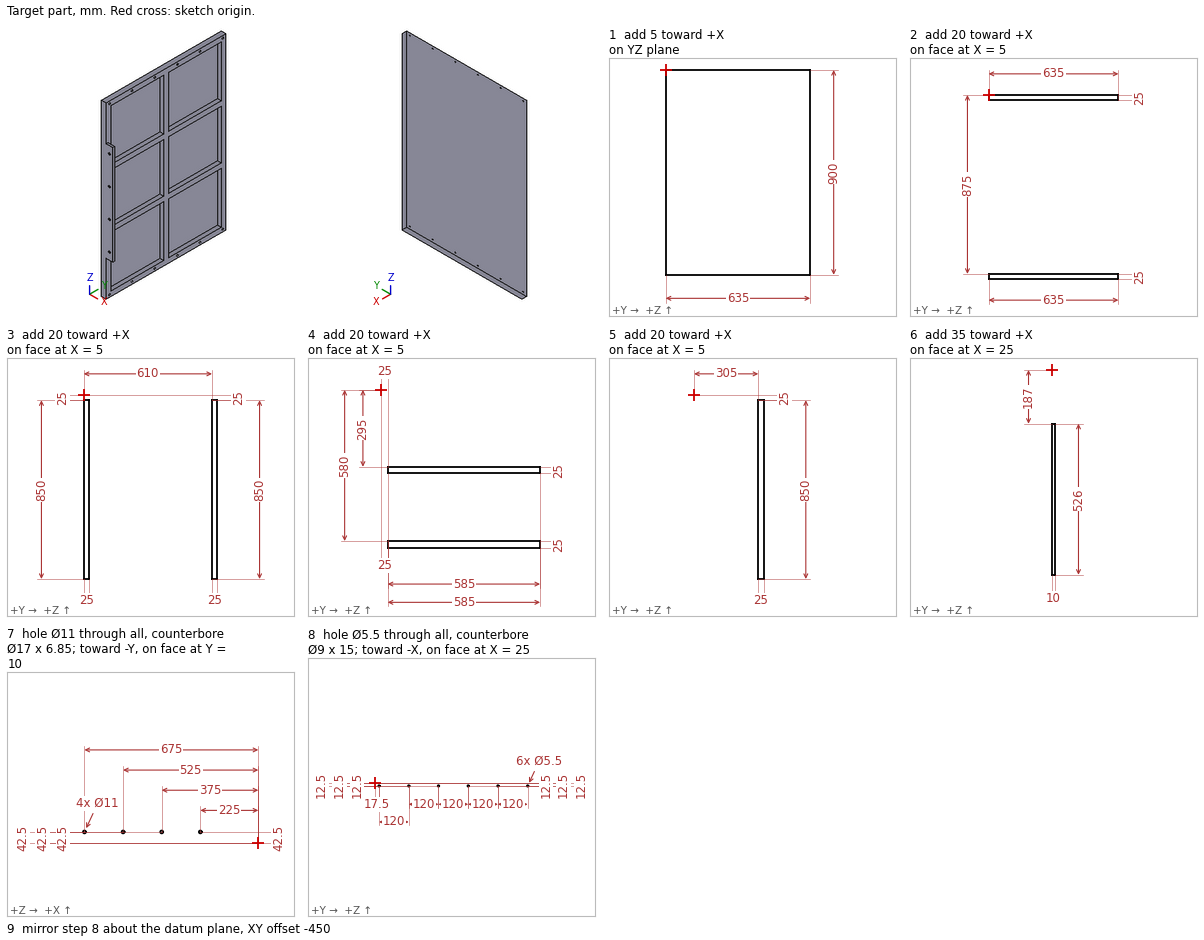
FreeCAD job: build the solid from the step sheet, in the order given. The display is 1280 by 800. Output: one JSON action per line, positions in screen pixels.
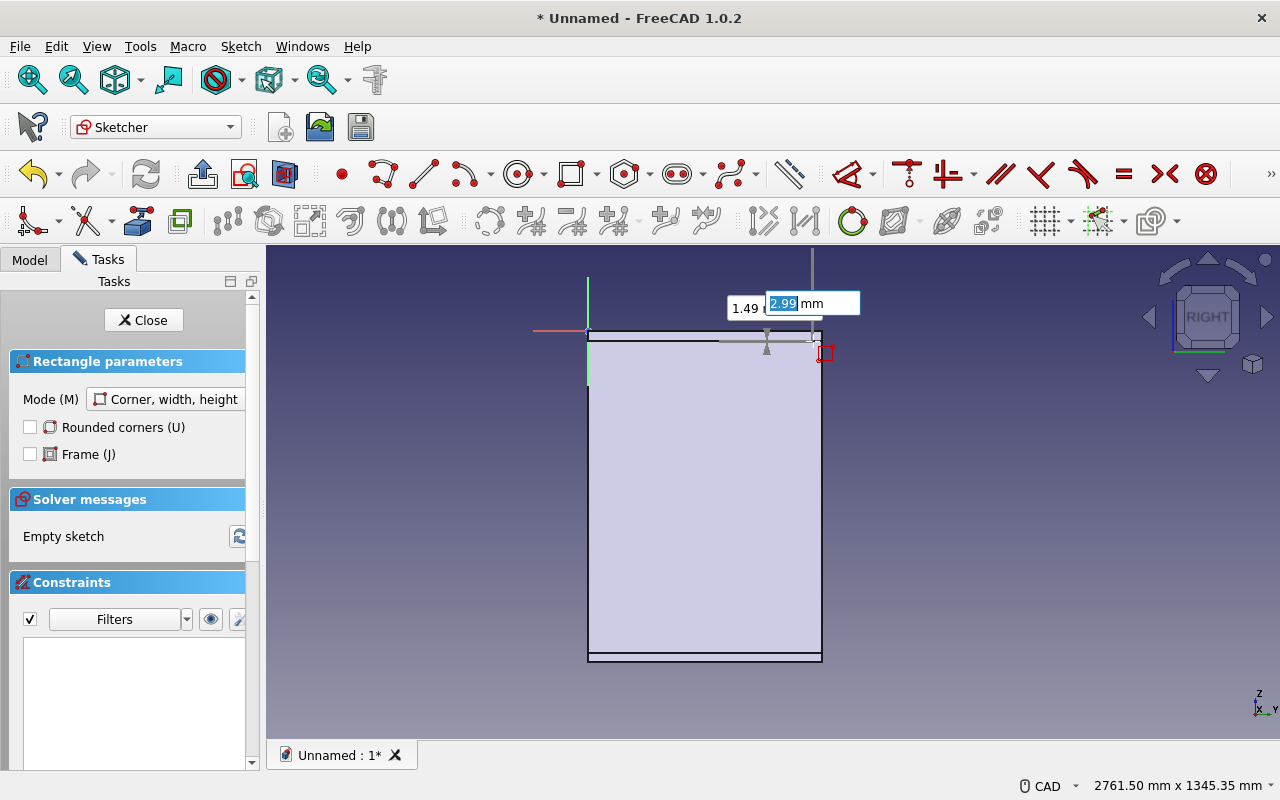
{"action": "left_click", "coordinate": [822, 653]}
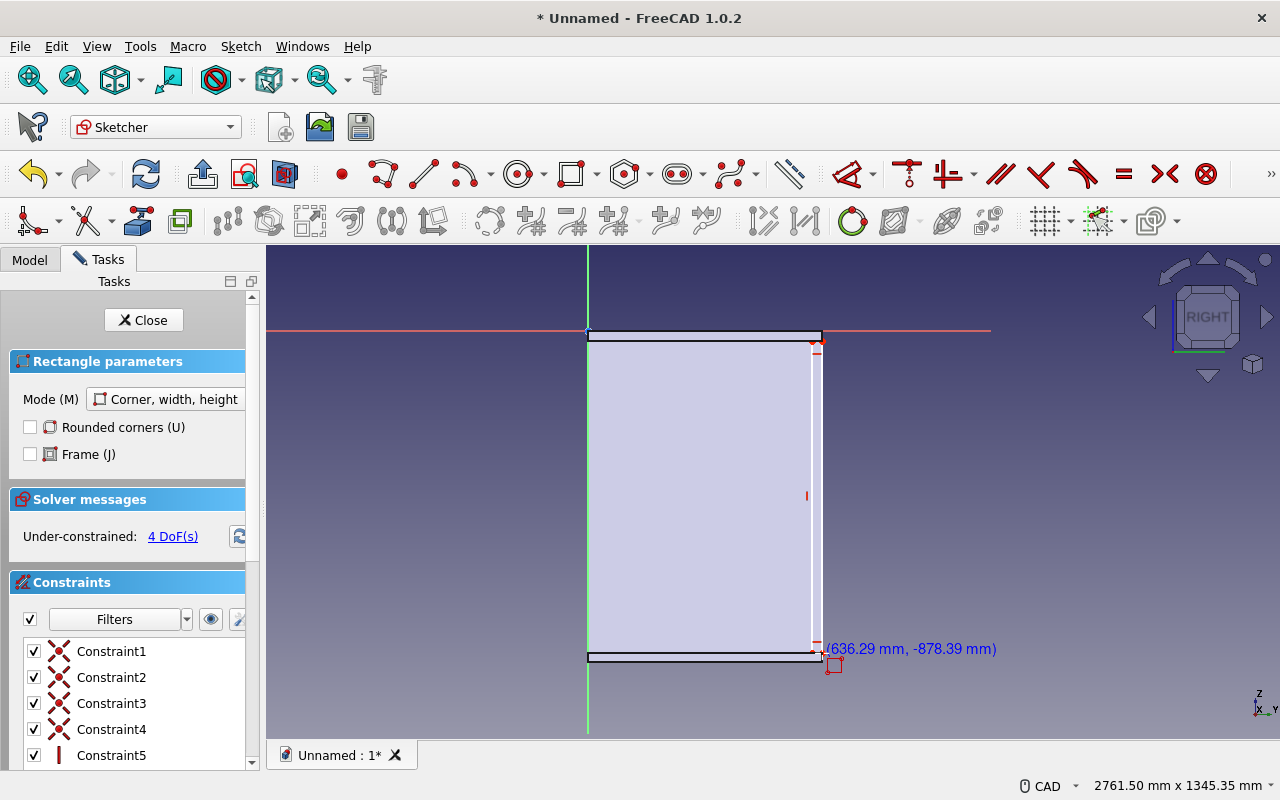
{"action": "scroll", "coordinate": [588, 341], "scroll_direction": "up", "scroll_amount": 3}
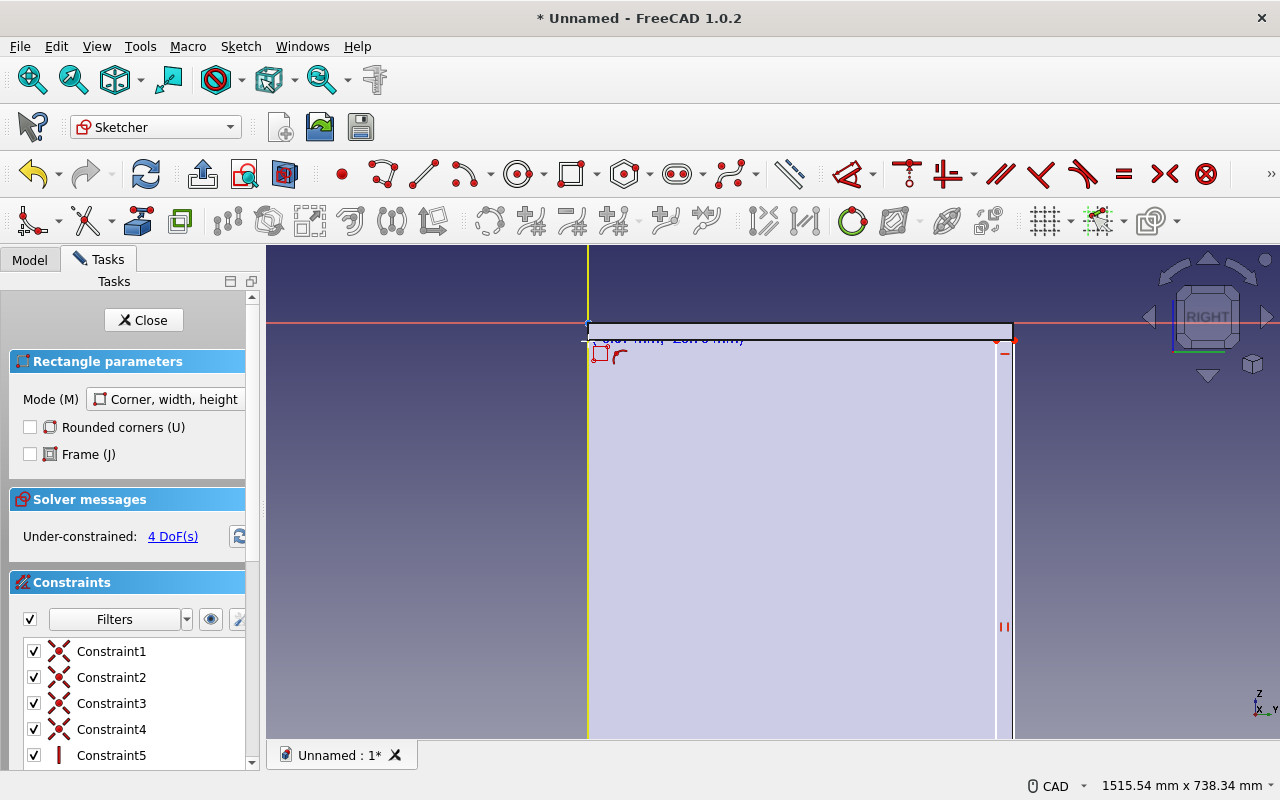
{"action": "left_click", "coordinate": [588, 340]}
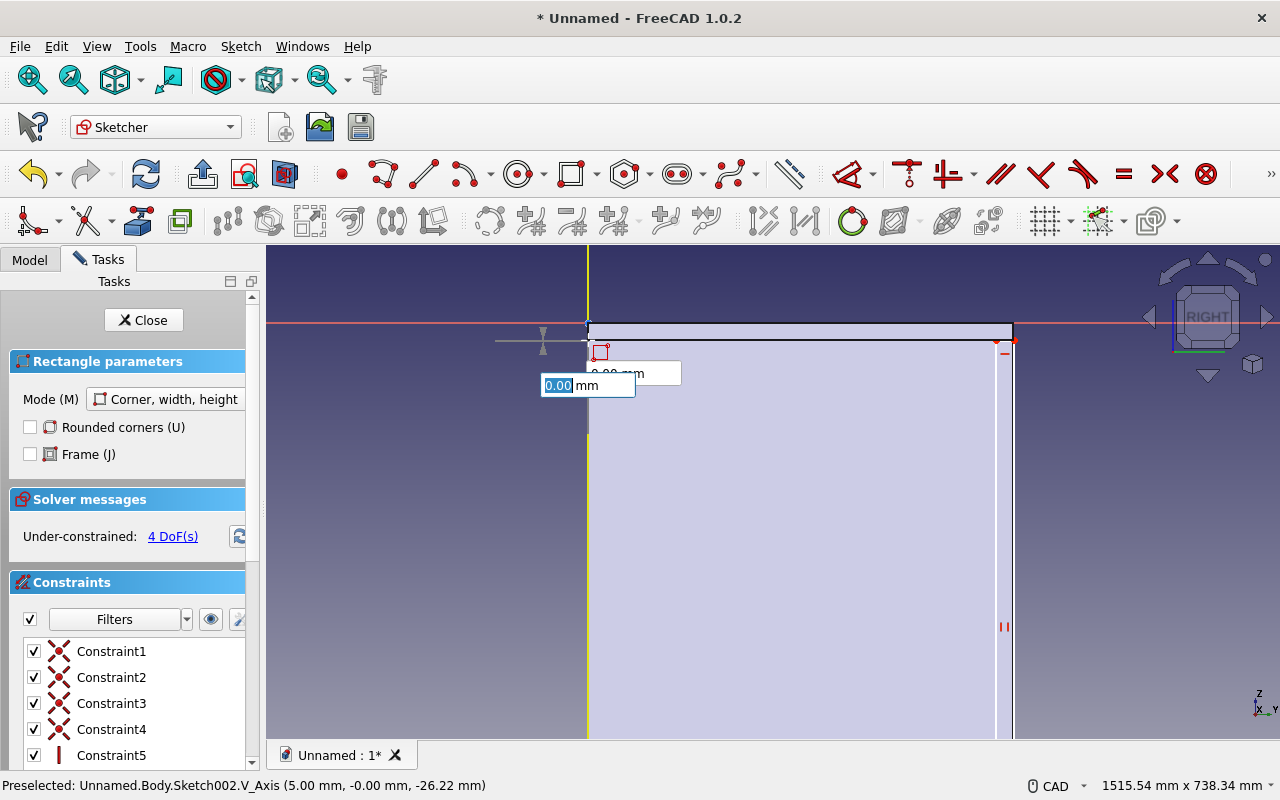
{"action": "scroll", "coordinate": [587, 341], "scroll_direction": "down", "scroll_amount": 3}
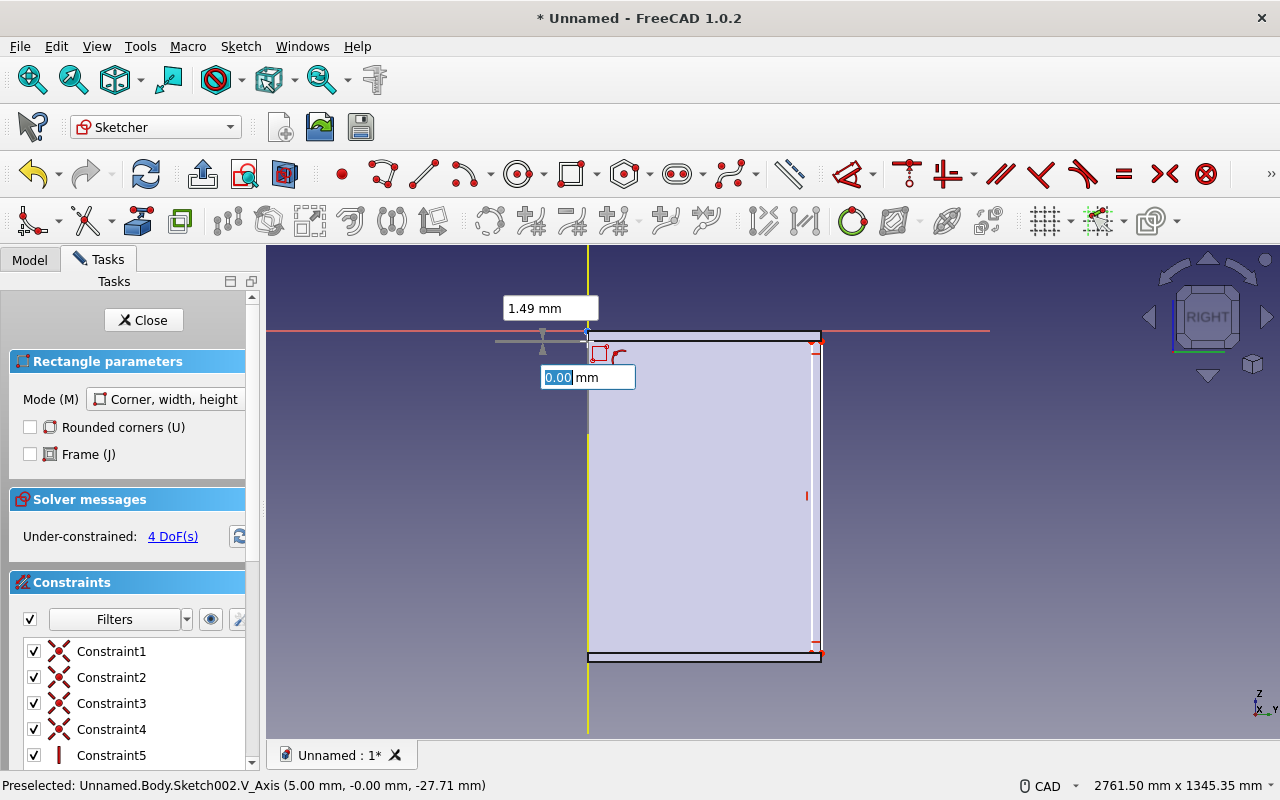
{"action": "scroll", "coordinate": [597, 653], "scroll_direction": "up", "scroll_amount": 3}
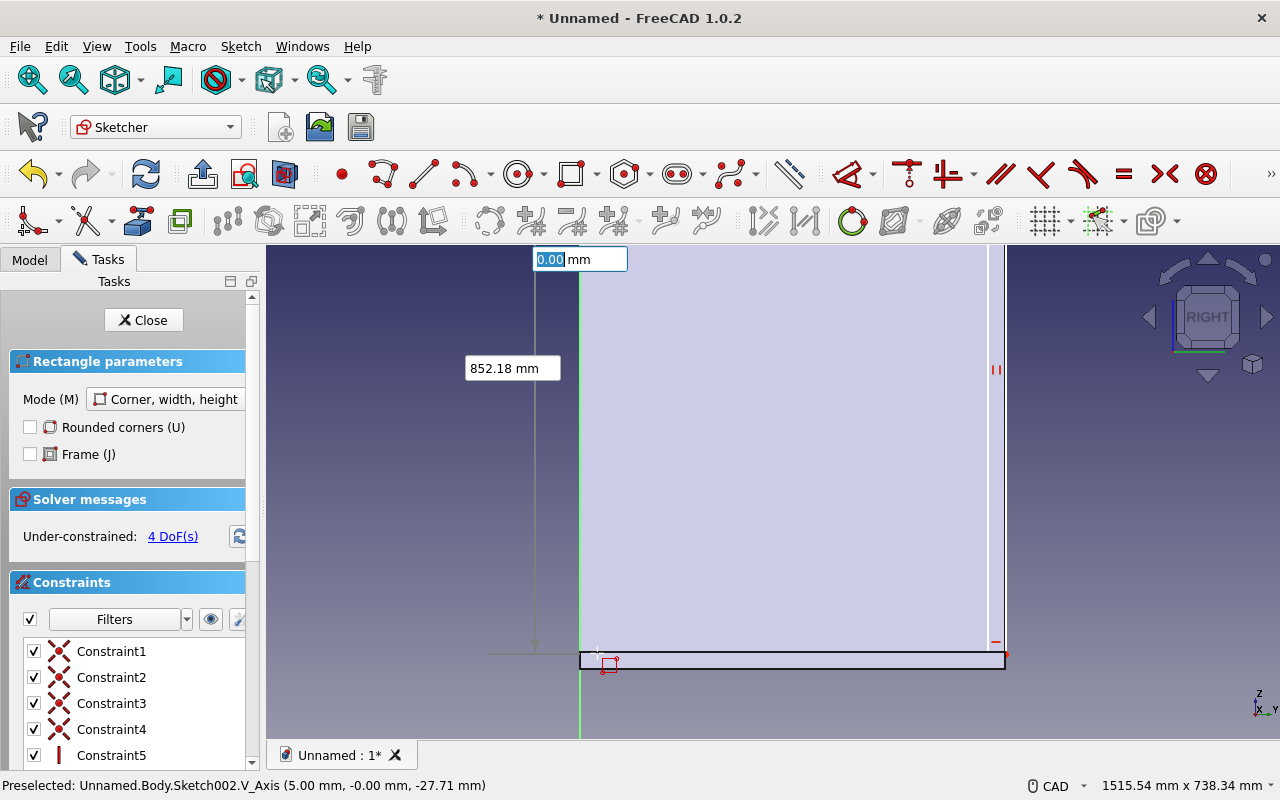
{"action": "left_click", "coordinate": [597, 652]}
{"action": "key", "text": "Escape"}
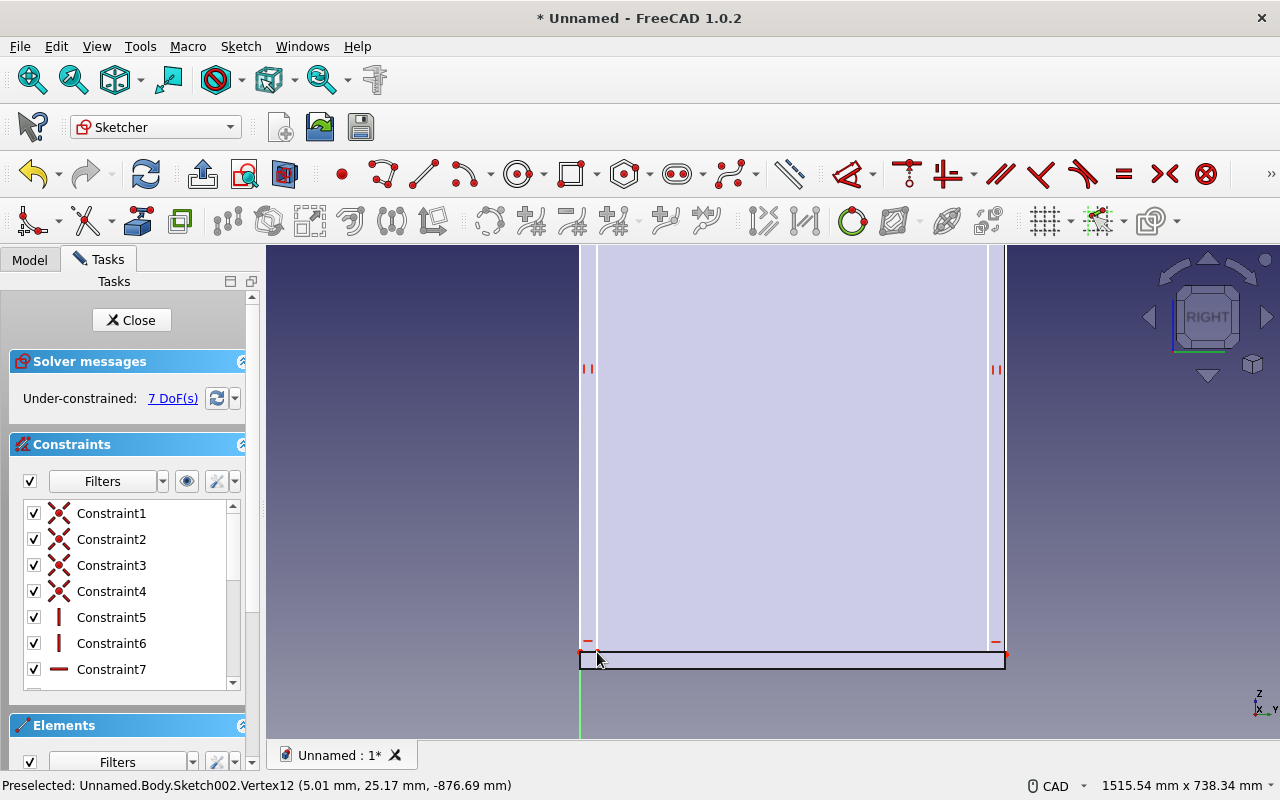
{"action": "left_click", "coordinate": [846, 174]}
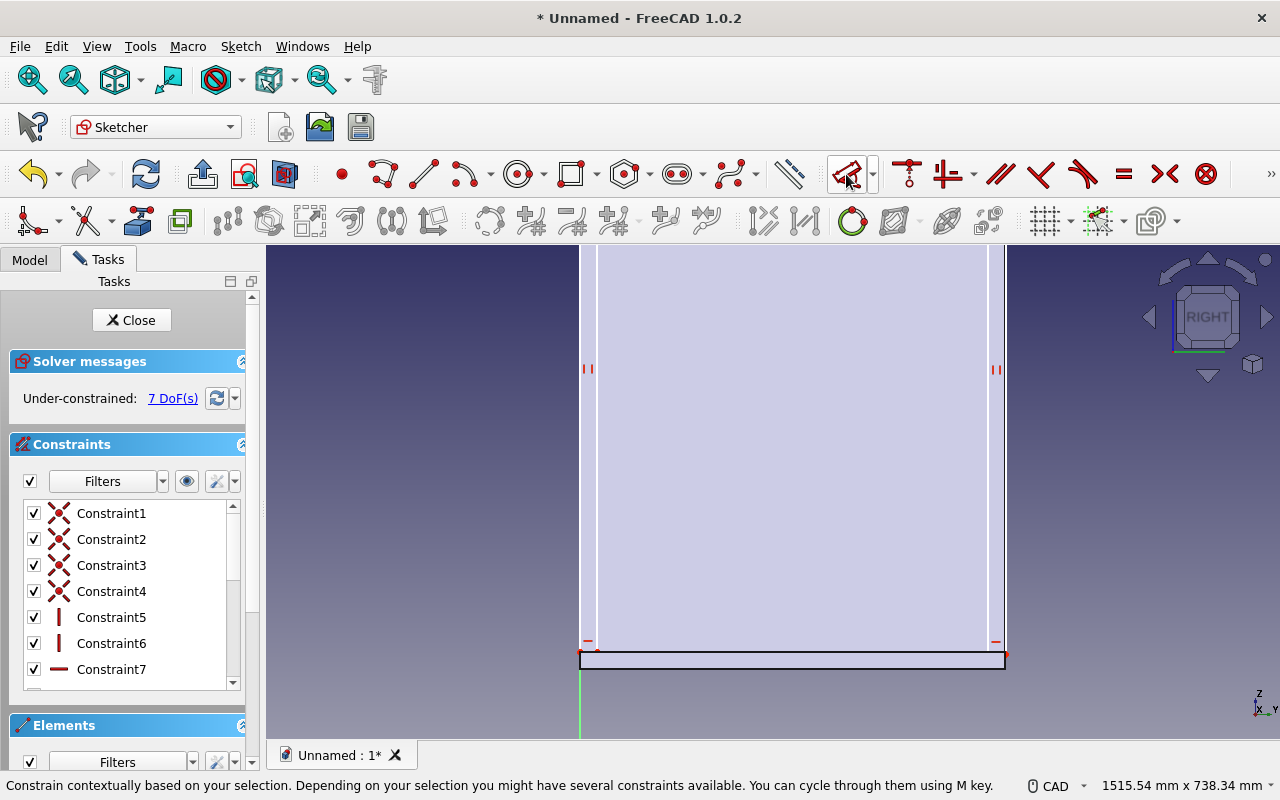
{"action": "scroll", "coordinate": [997, 654], "scroll_direction": "up", "scroll_amount": 5}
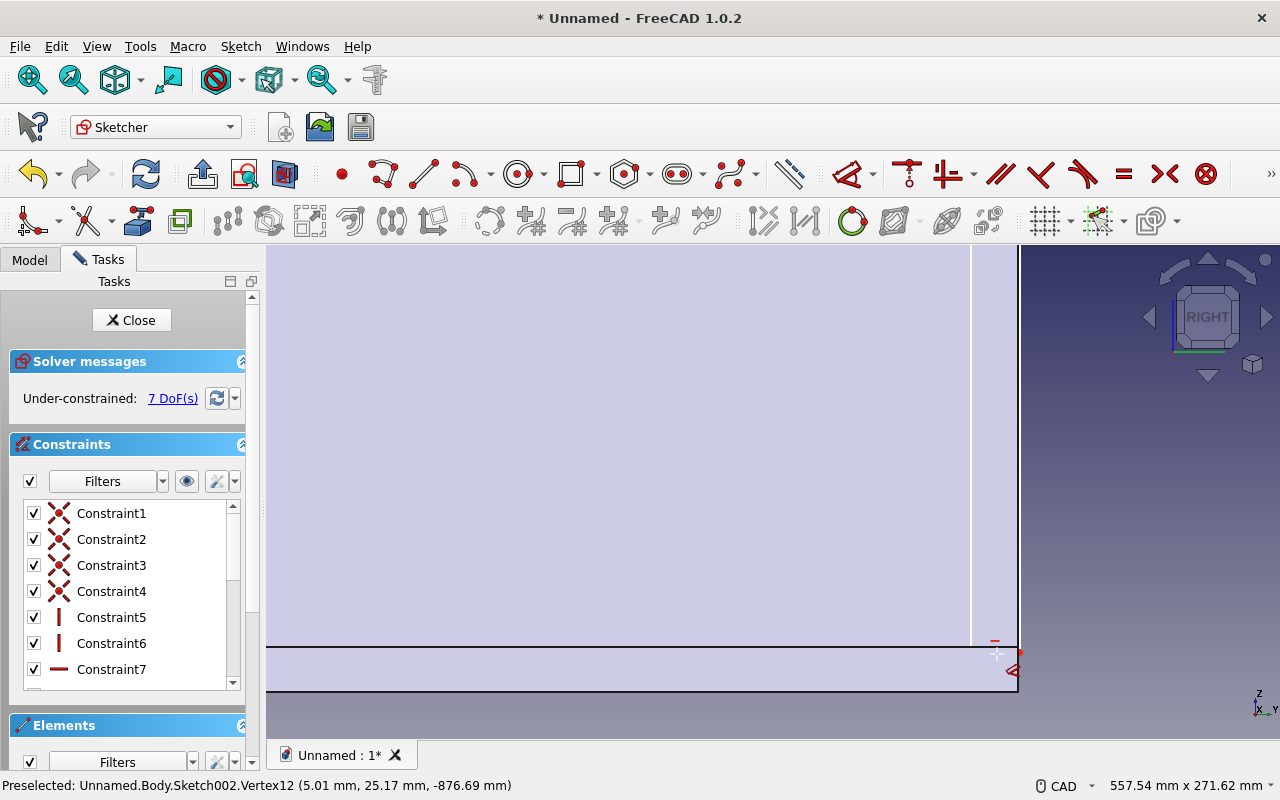
{"action": "left_click", "coordinate": [996, 653]}
{"action": "left_click", "coordinate": [996, 687]}